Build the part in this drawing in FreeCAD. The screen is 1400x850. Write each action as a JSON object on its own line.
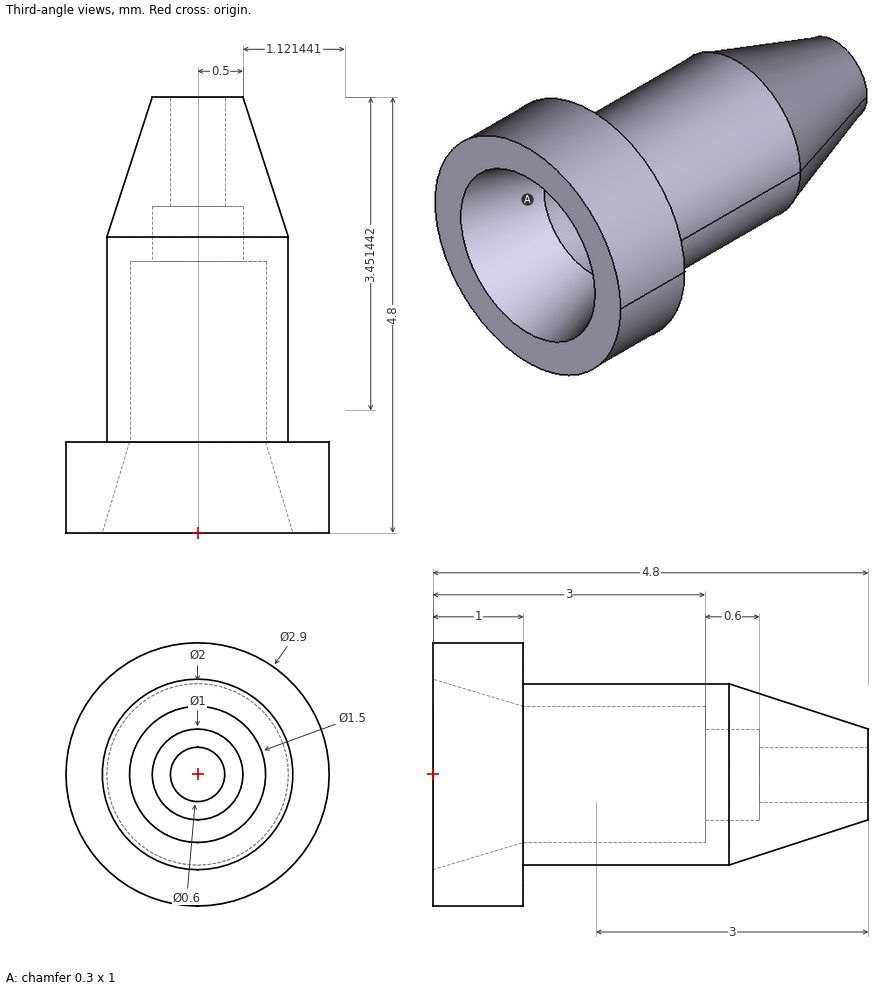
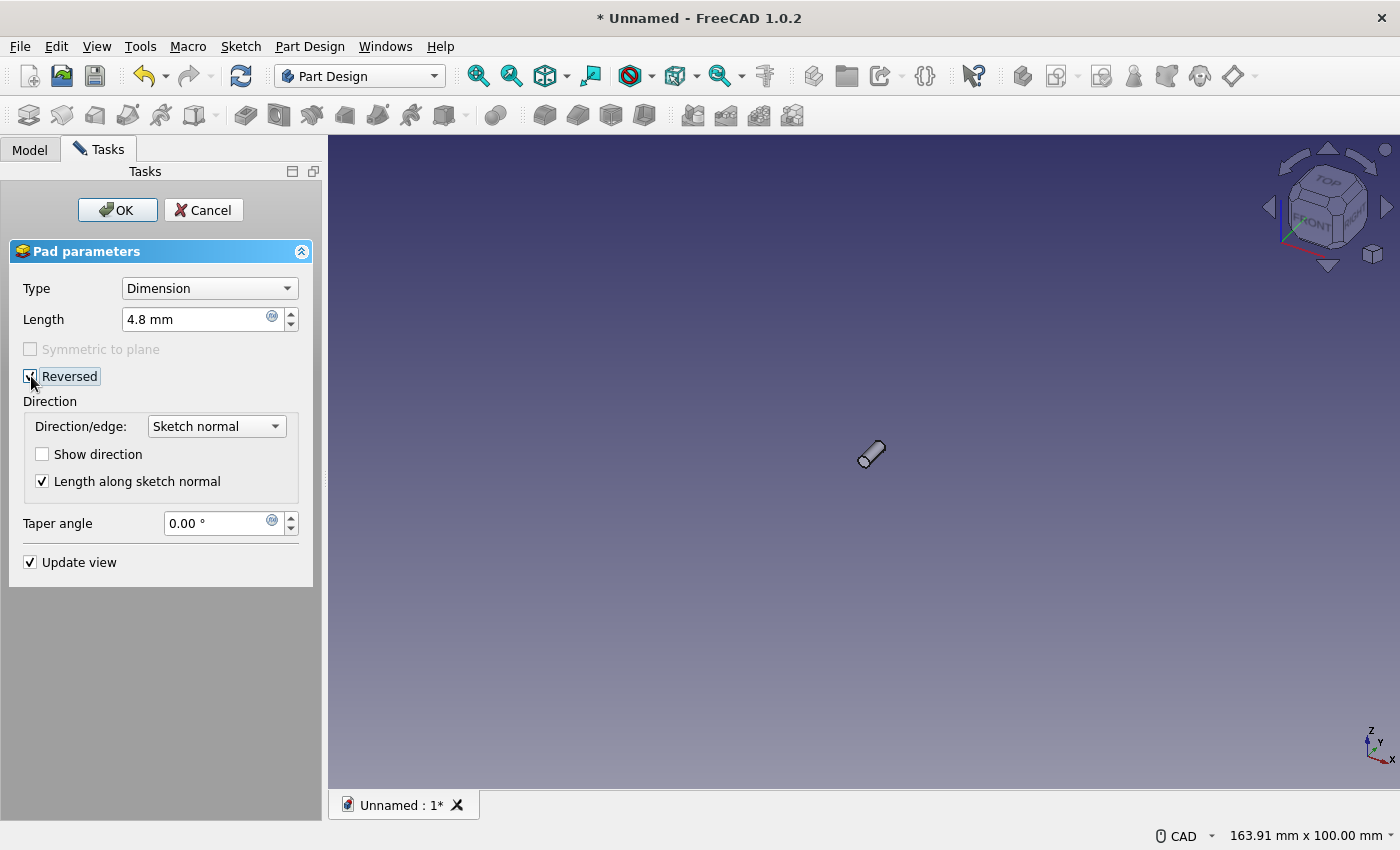
{"action": "left_click", "coordinate": [118, 210]}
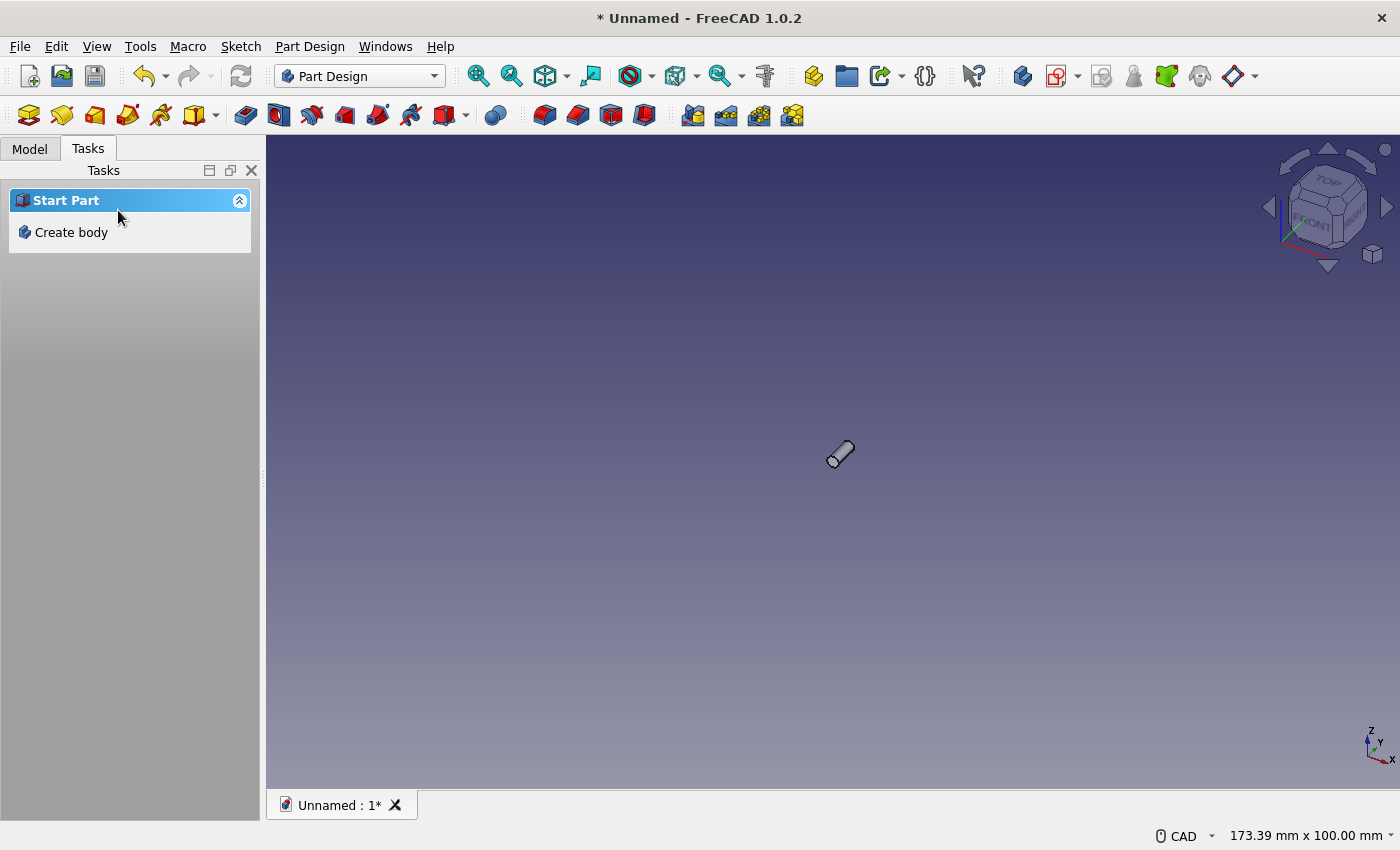
{"action": "left_click", "coordinate": [479, 76]}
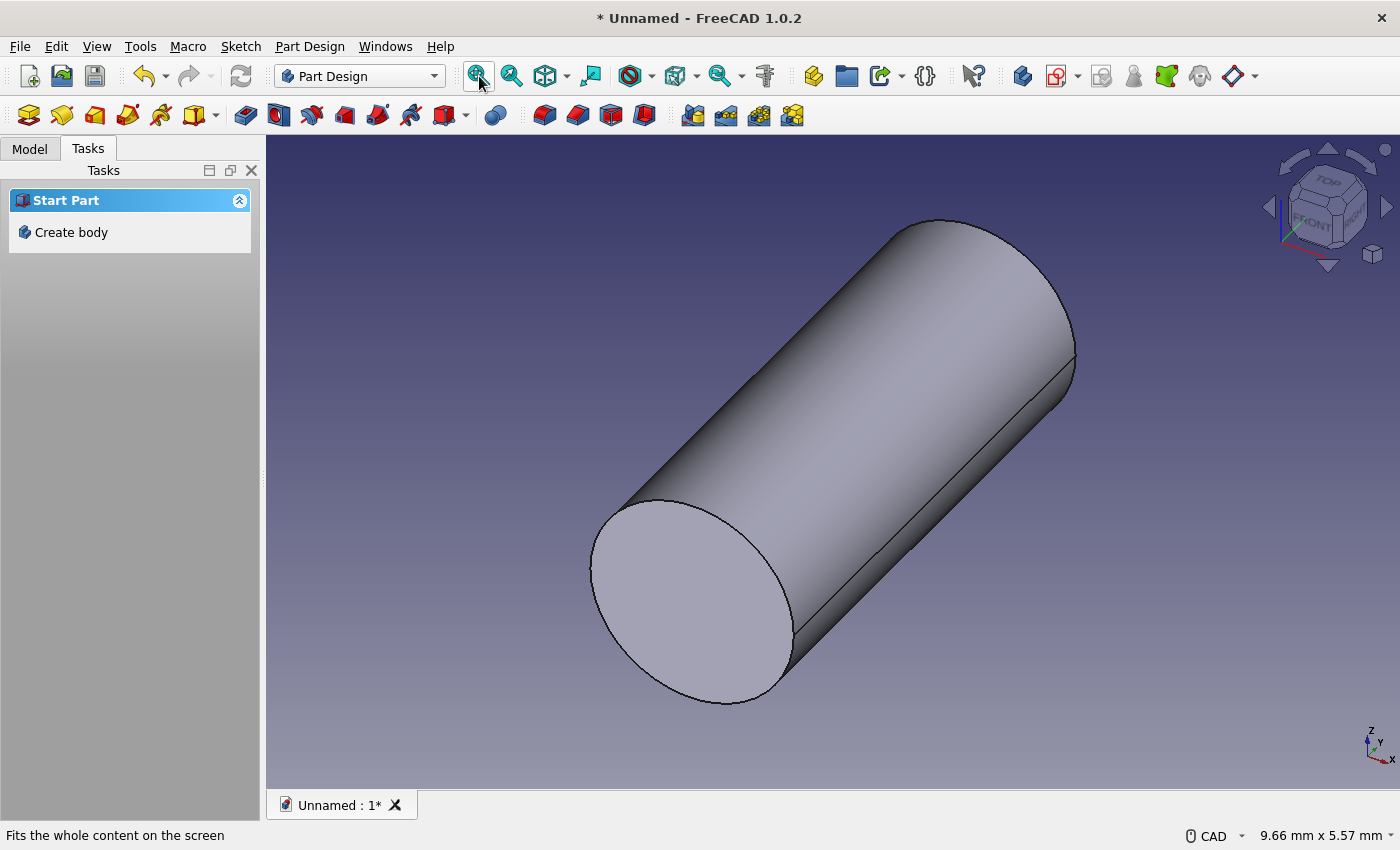
{"action": "left_click", "coordinate": [1056, 76]}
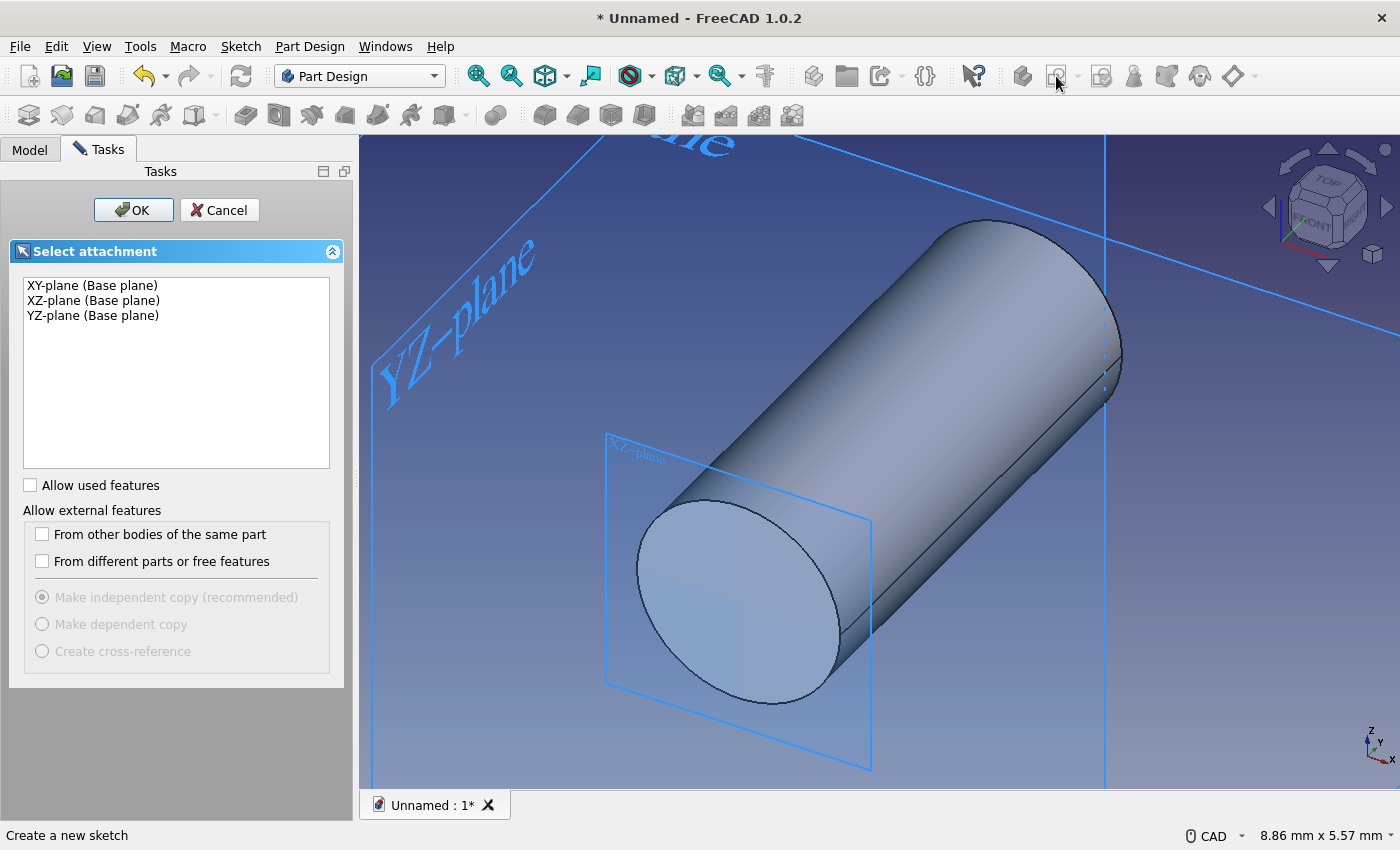
{"action": "left_click", "coordinate": [84, 286]}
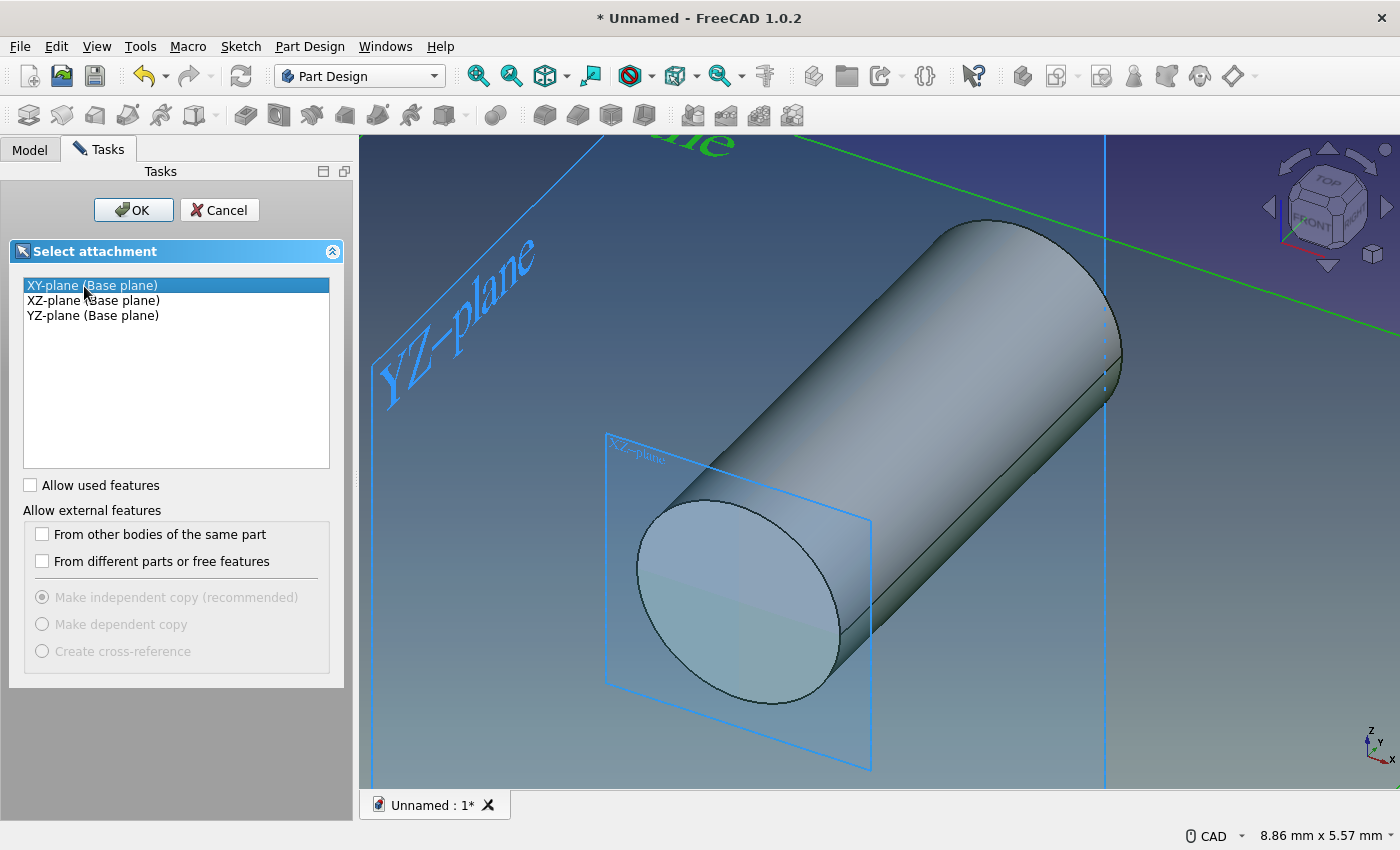
{"action": "left_click", "coordinate": [134, 210]}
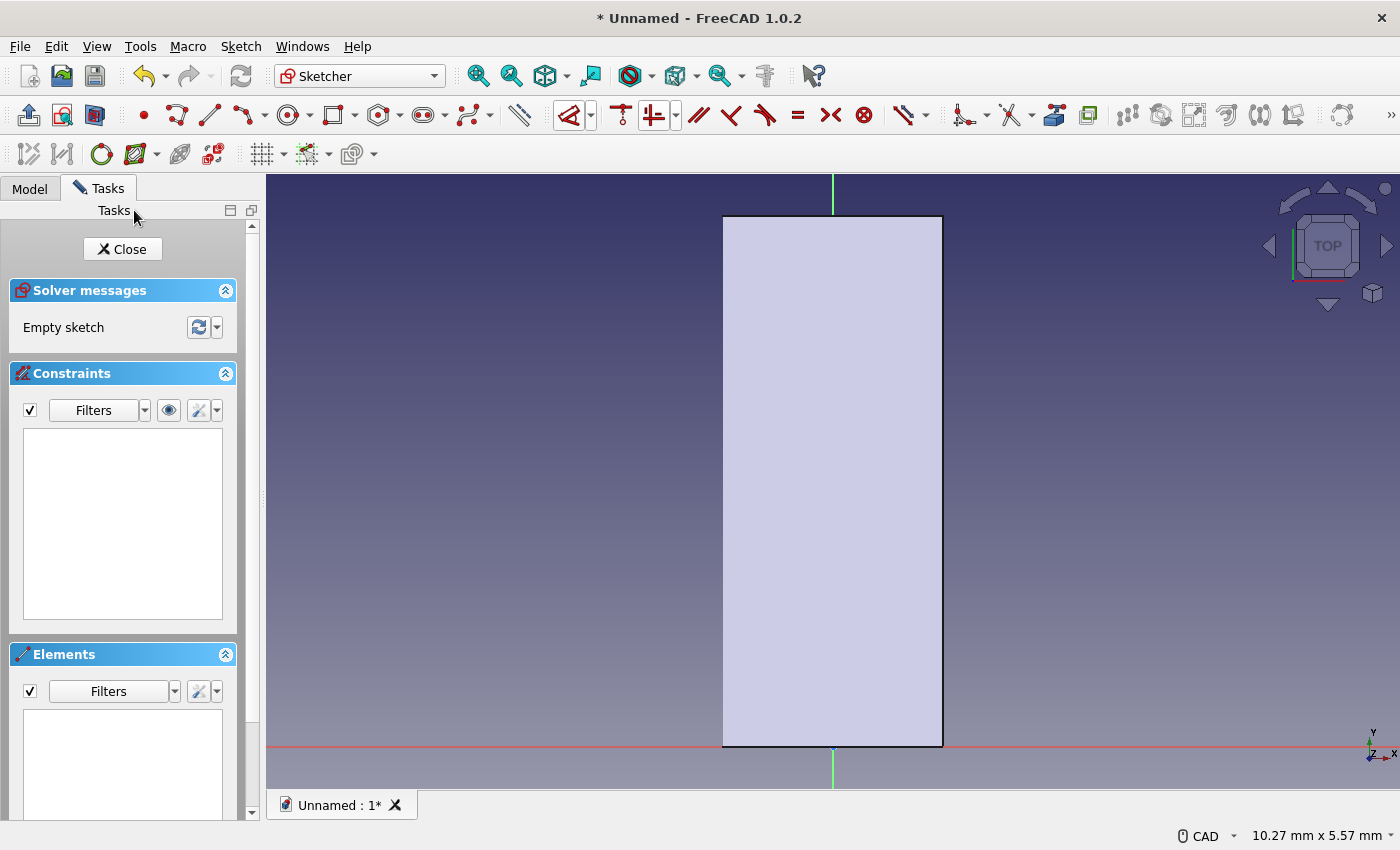
{"action": "left_click", "coordinate": [95, 116]}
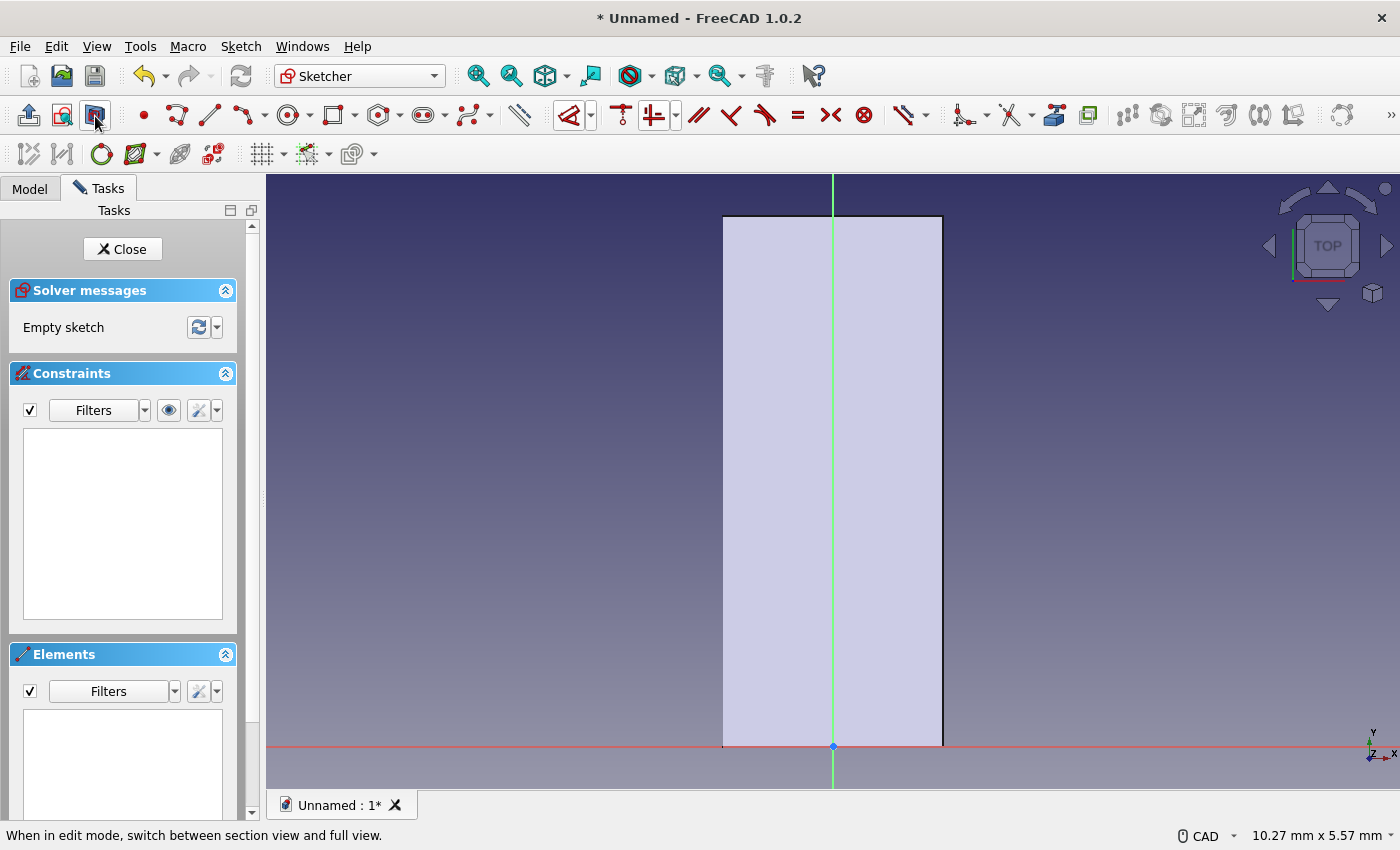
{"action": "scroll", "coordinate": [294, 481], "scroll_direction": "down", "scroll_amount": 1}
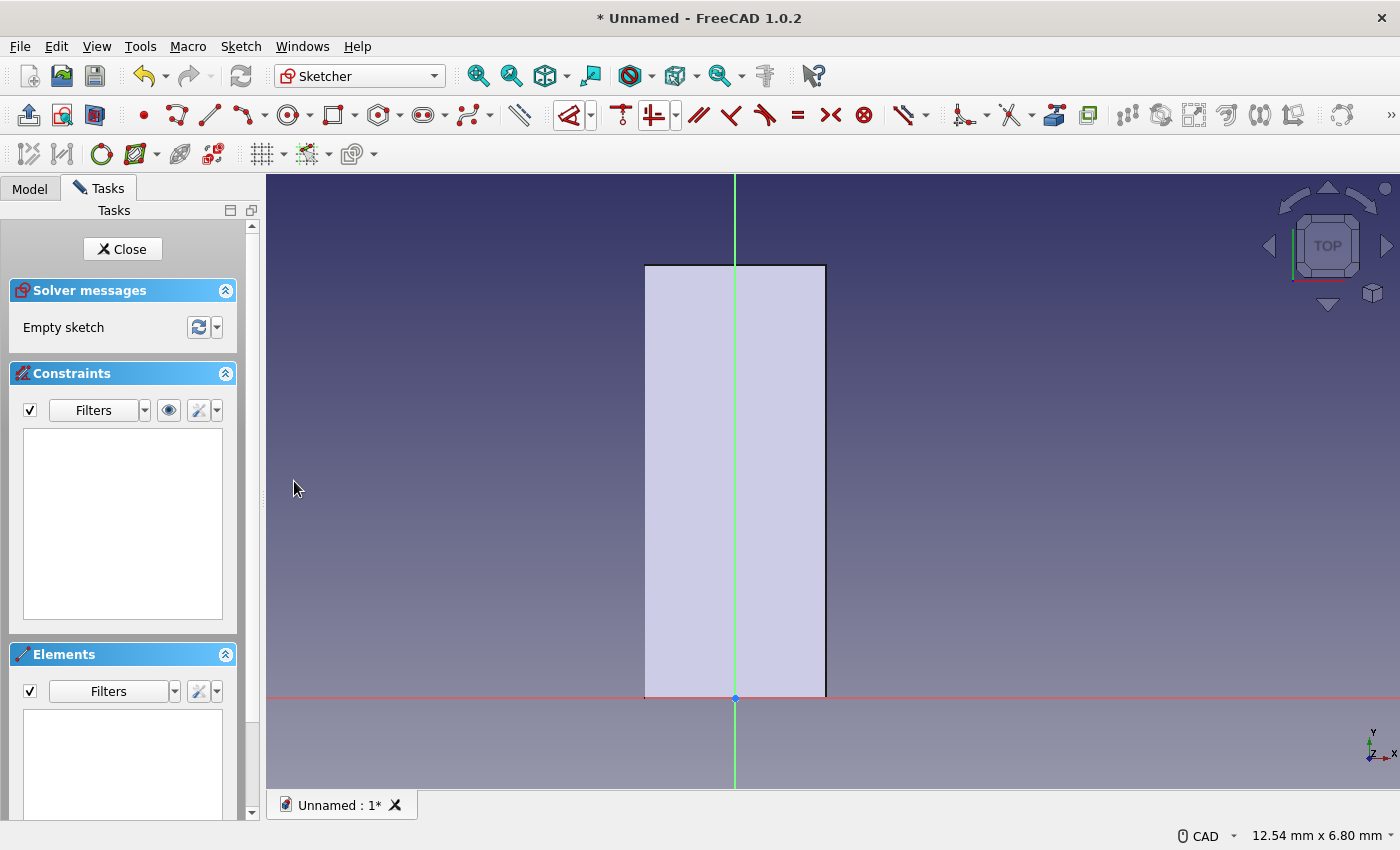
{"action": "key", "text": "g m"}